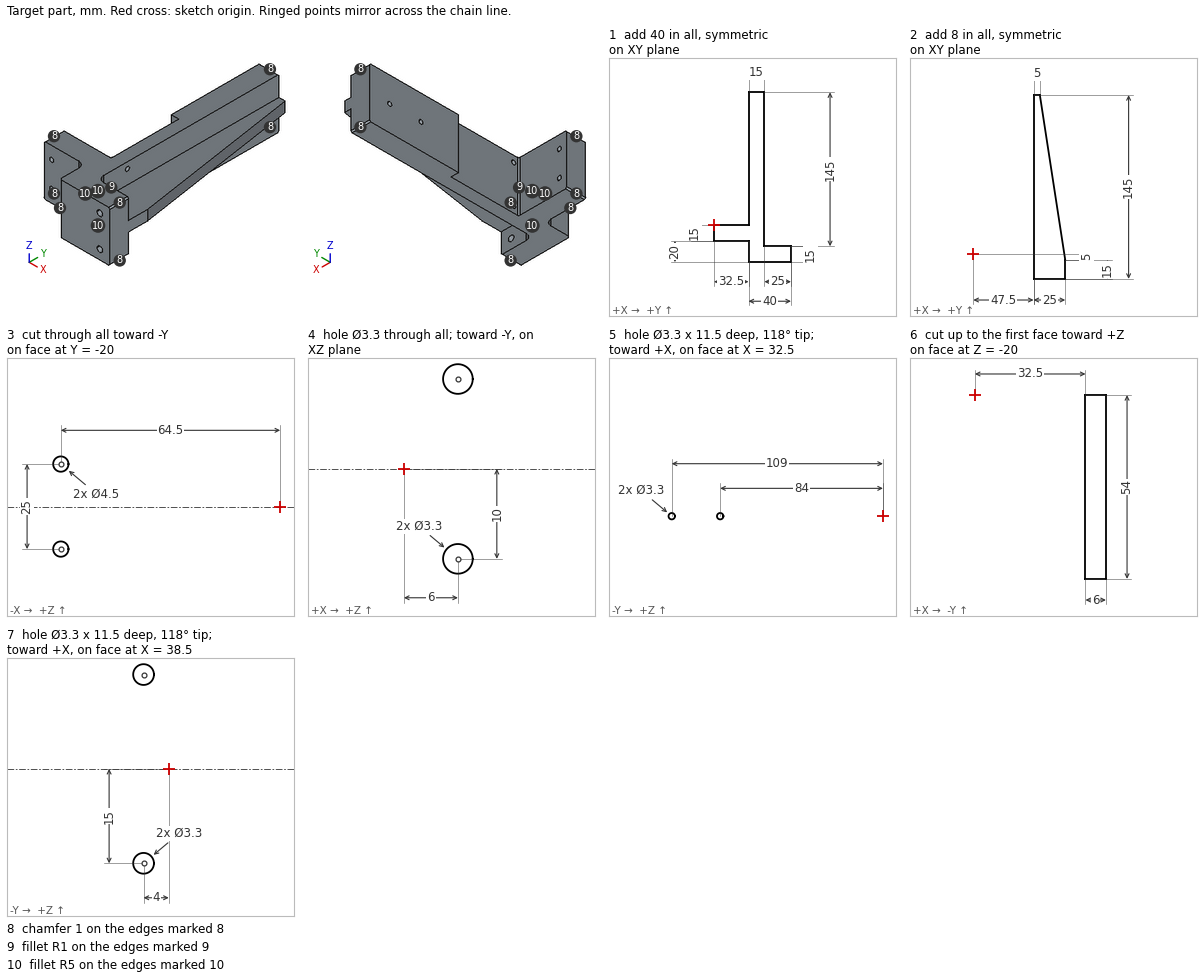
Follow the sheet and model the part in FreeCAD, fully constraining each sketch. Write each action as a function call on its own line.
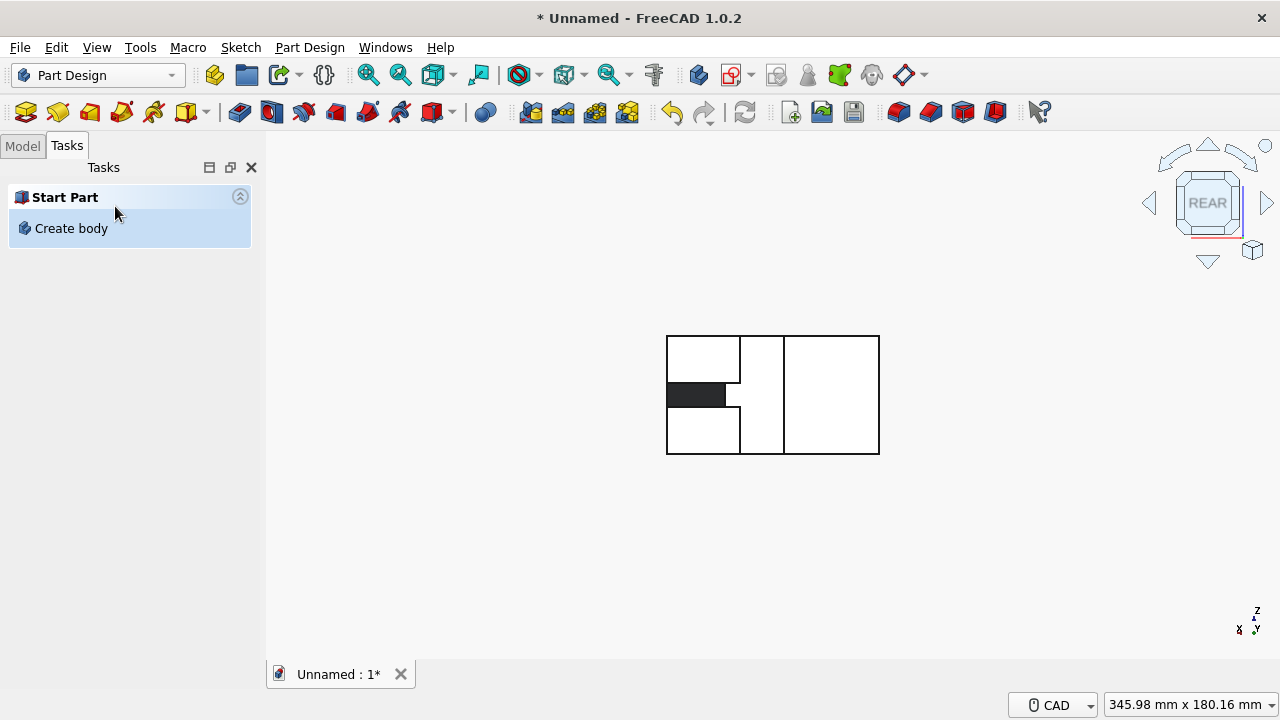
click(370, 76)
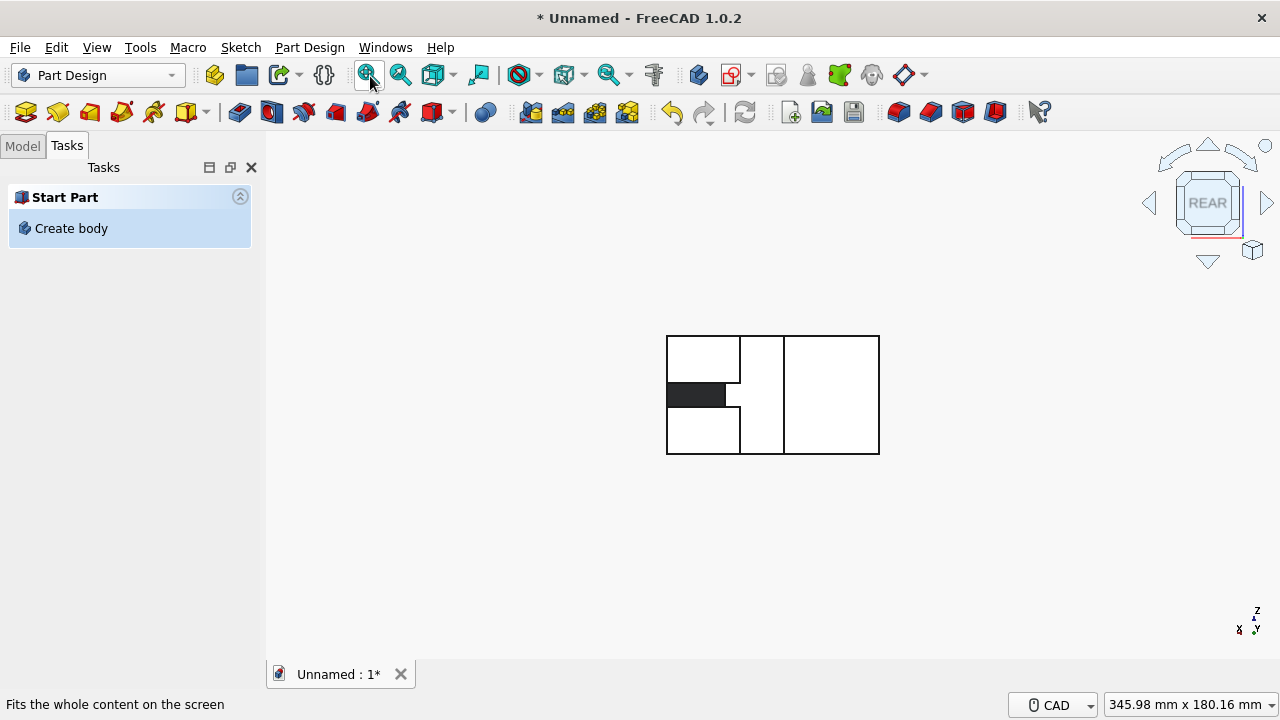
click(693, 429)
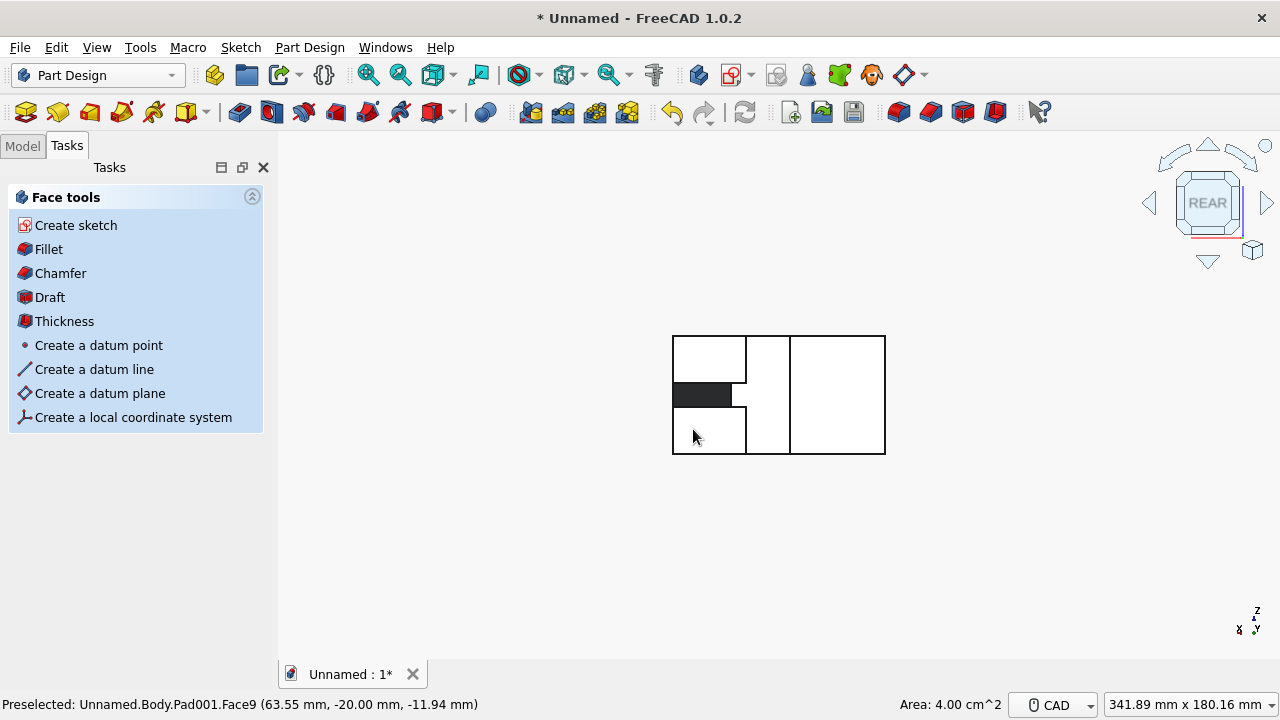
click(732, 76)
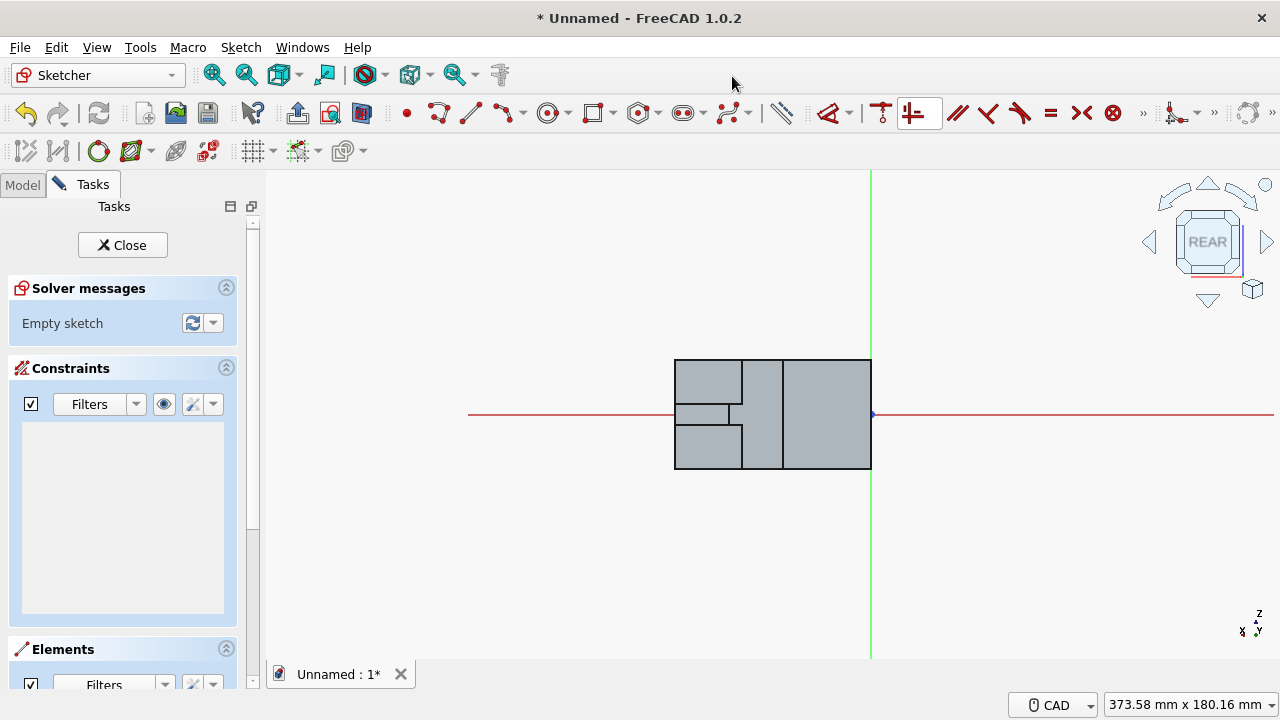
key(q)
key(s)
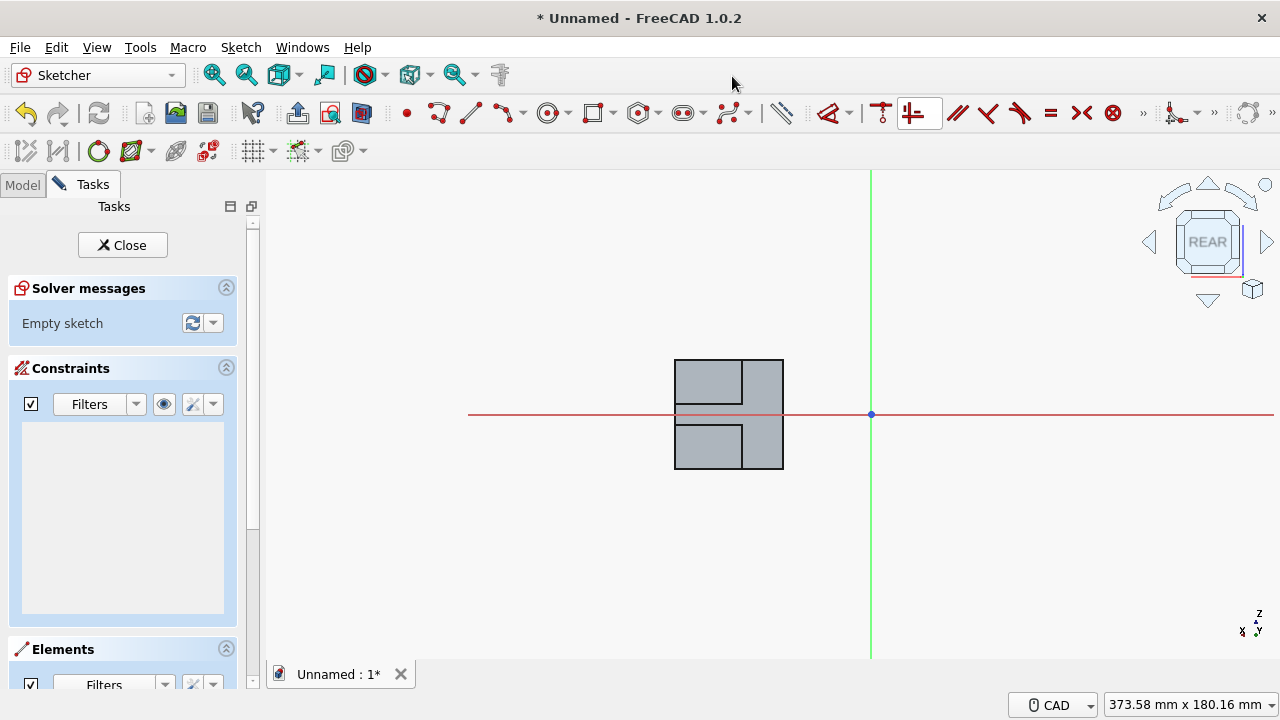
scroll(814, 415, up, 6)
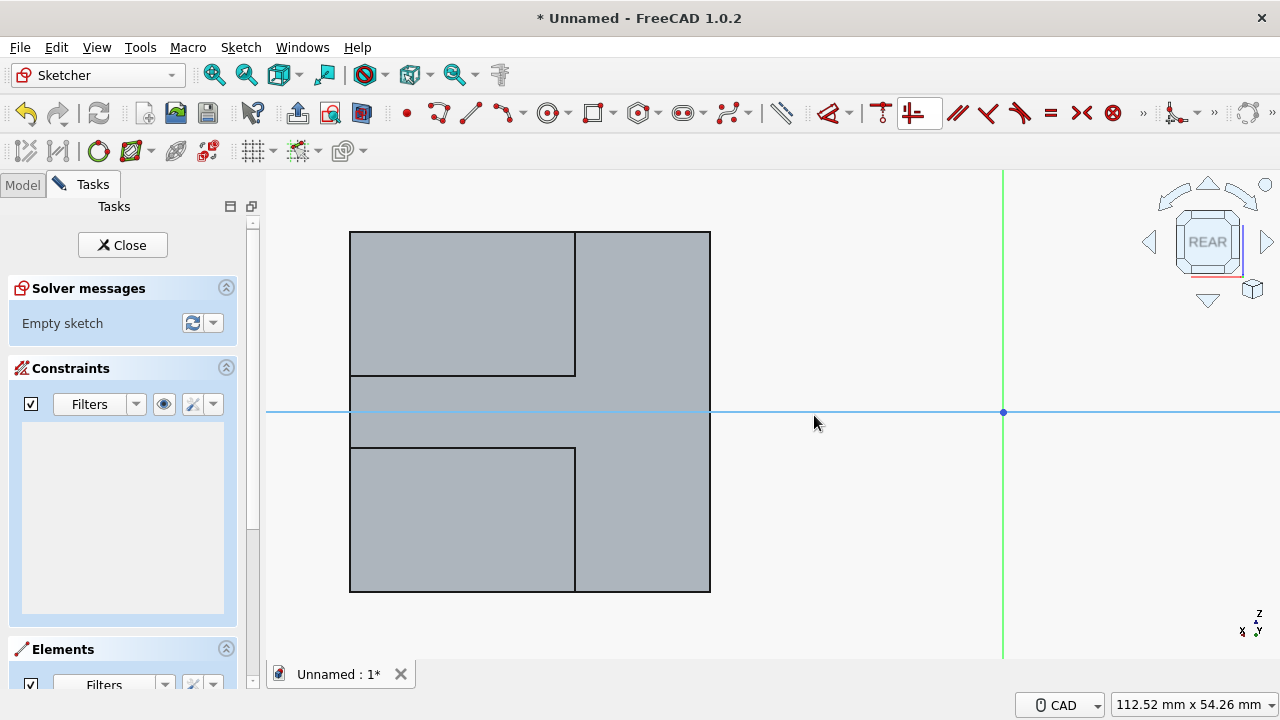
click(548, 114)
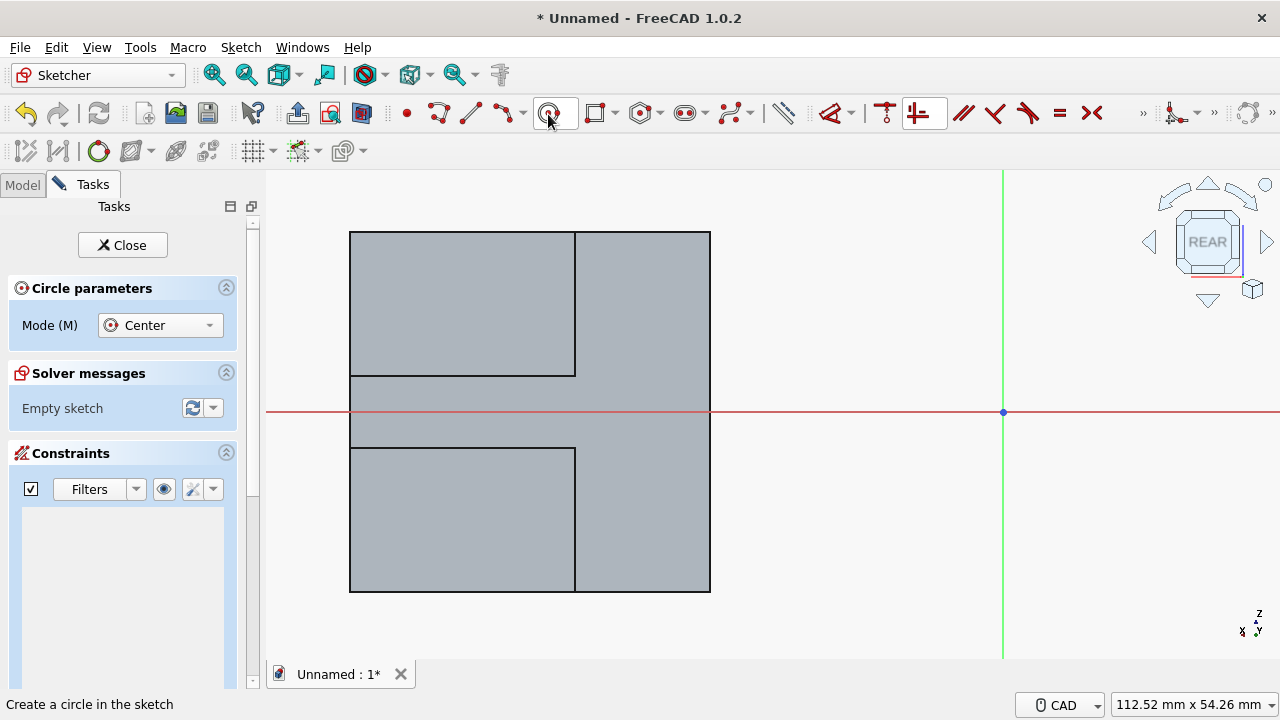
click(422, 300)
click(436, 285)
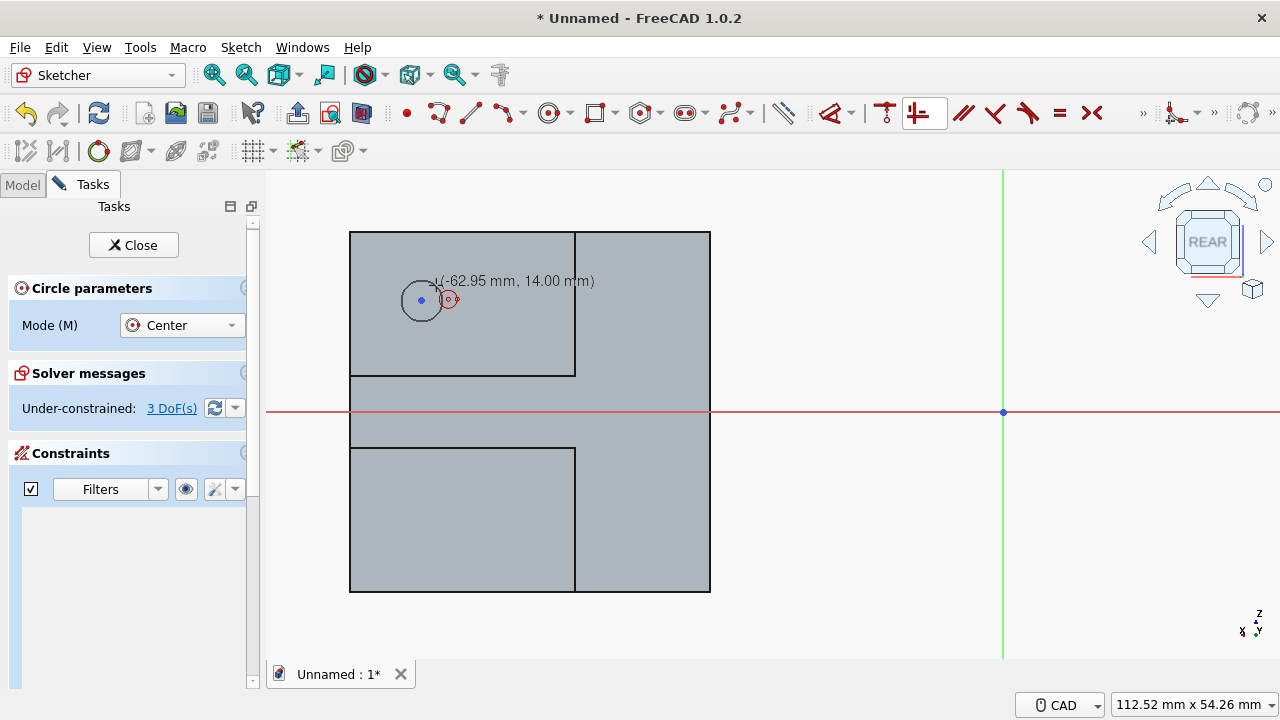
click(422, 525)
click(436, 510)
key(Escape)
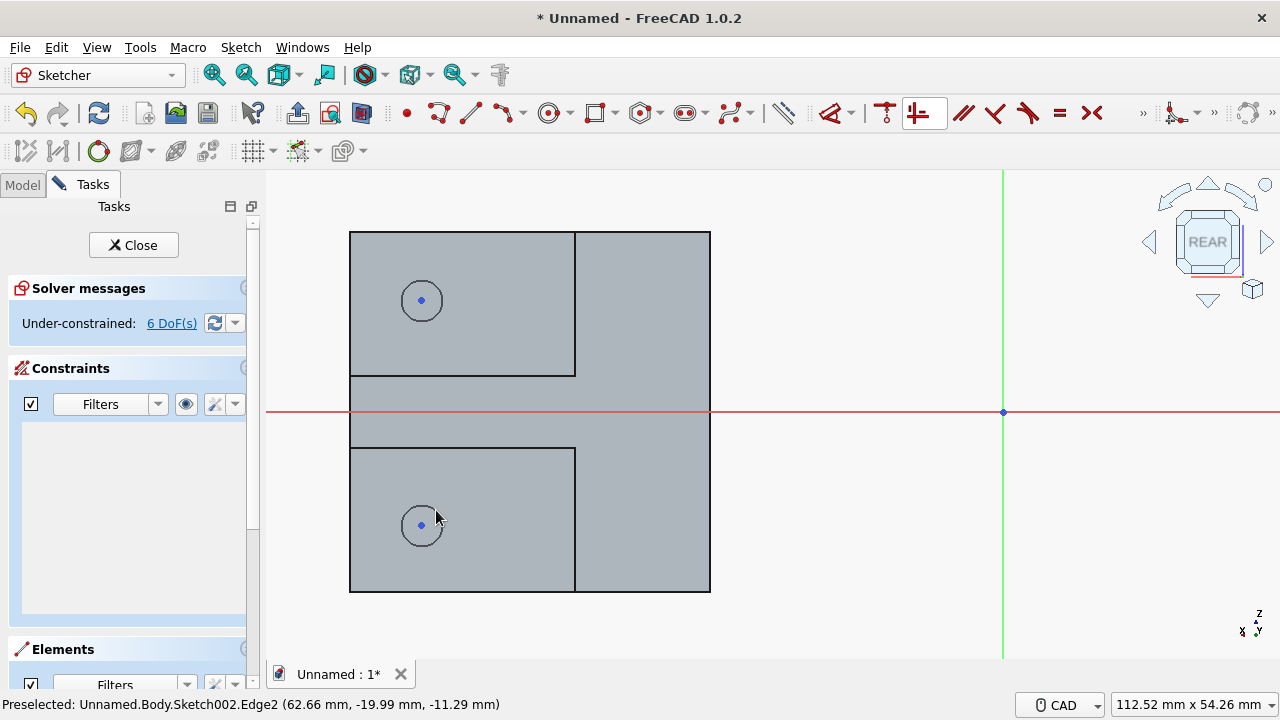
click(436, 286)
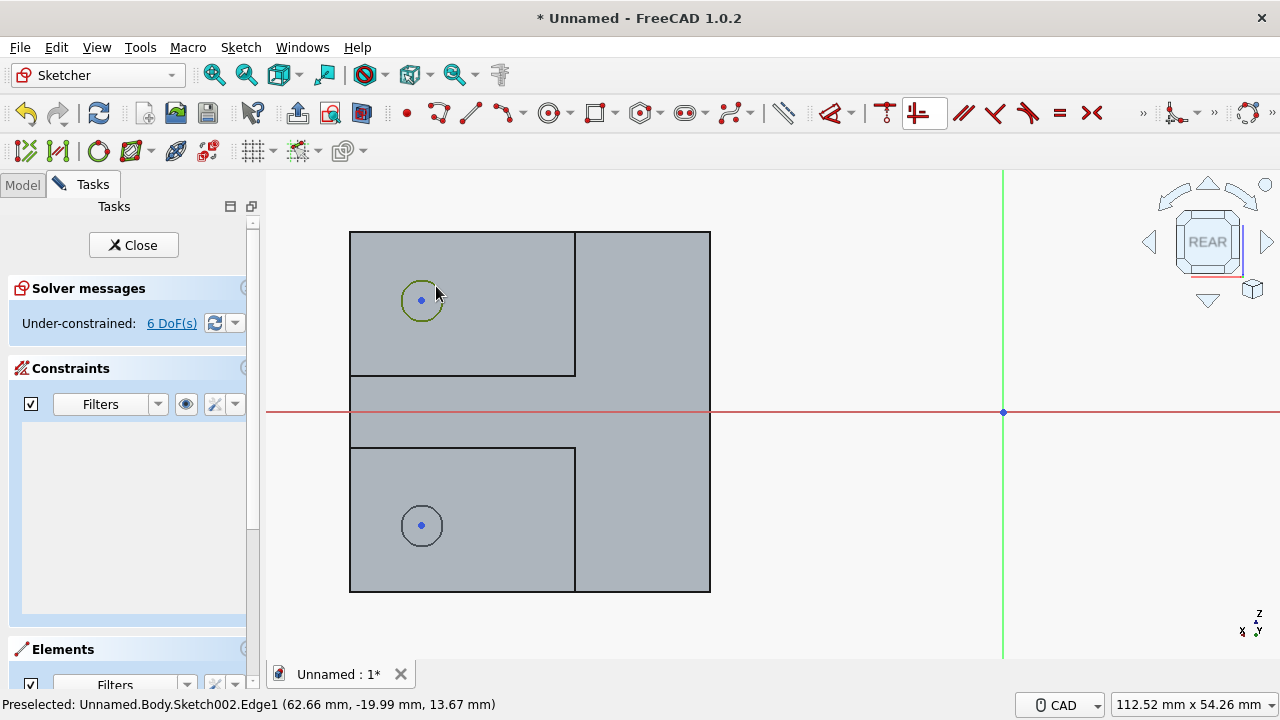
click(436, 511)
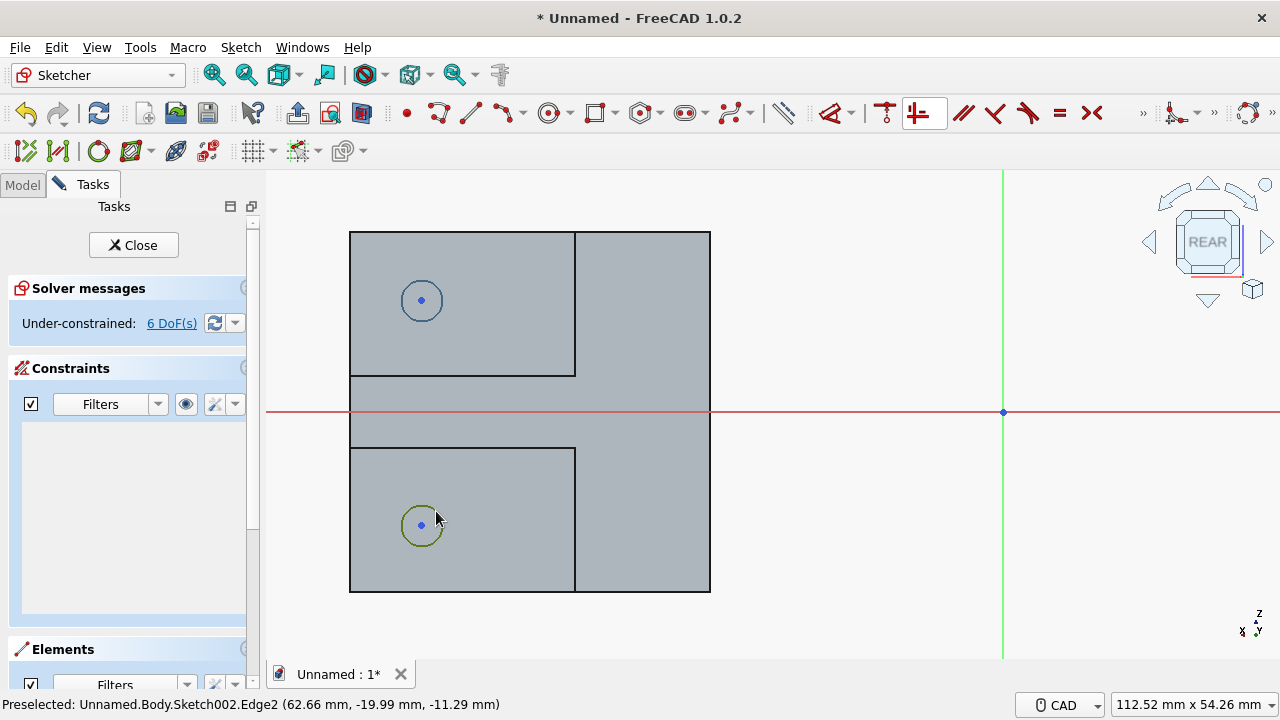
click(1060, 114)